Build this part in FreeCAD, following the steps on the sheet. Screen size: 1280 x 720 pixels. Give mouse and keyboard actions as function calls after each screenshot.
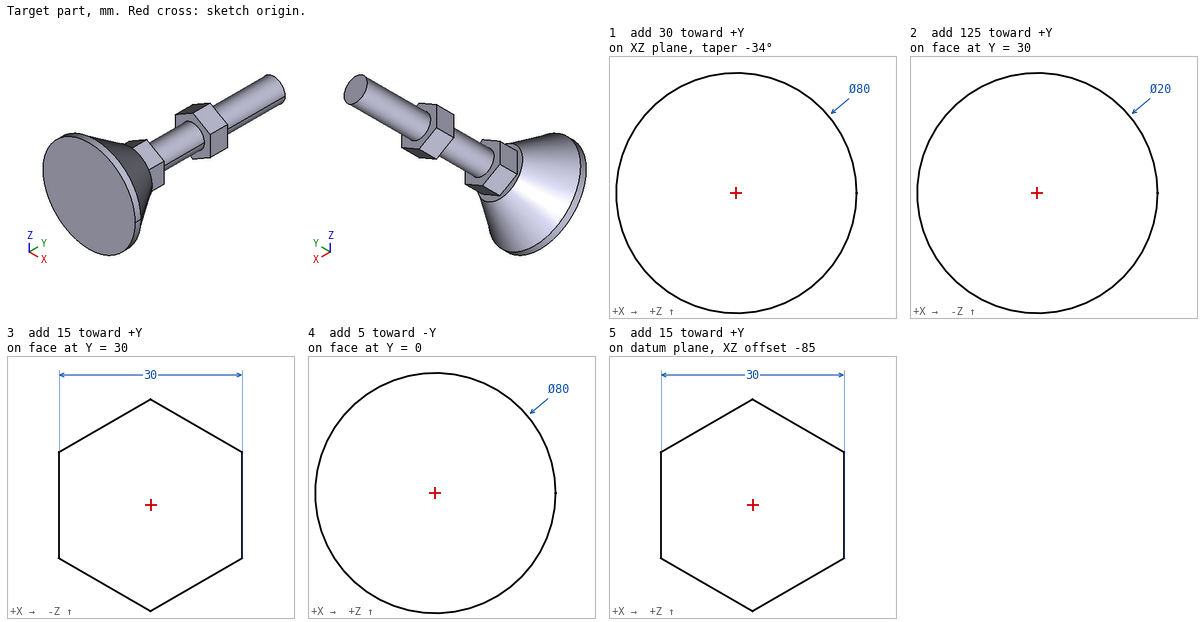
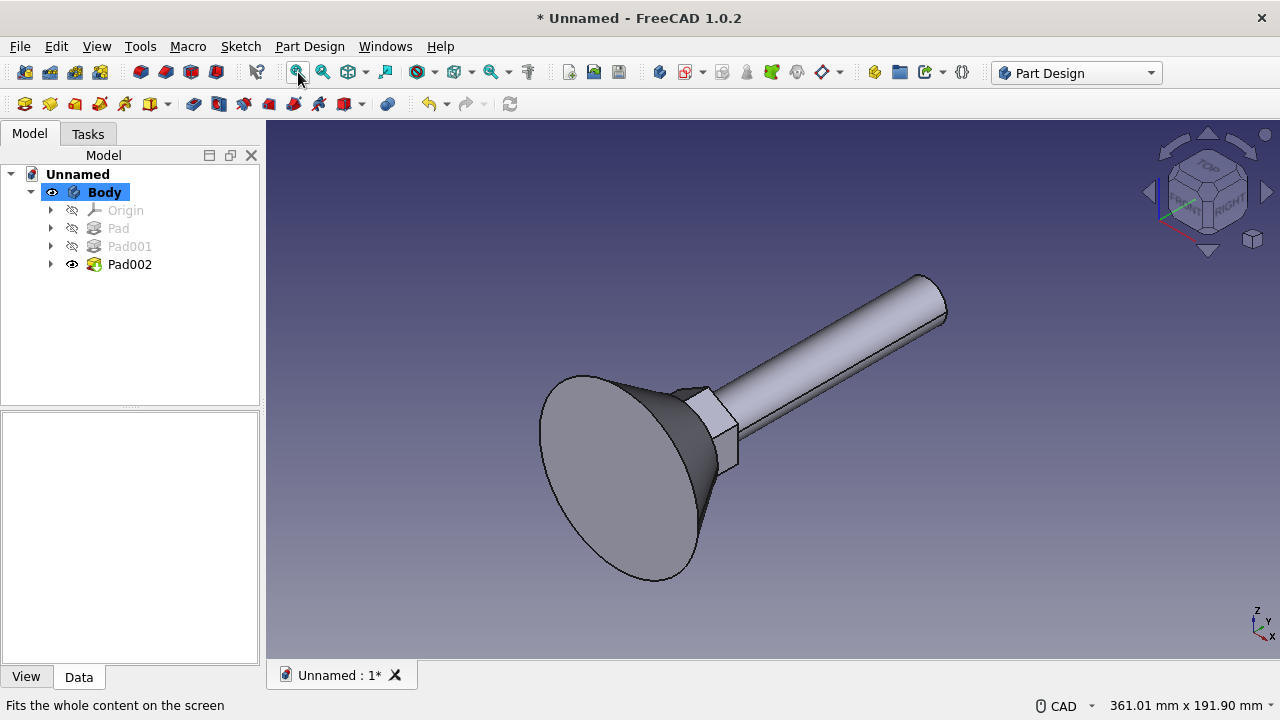
click(619, 477)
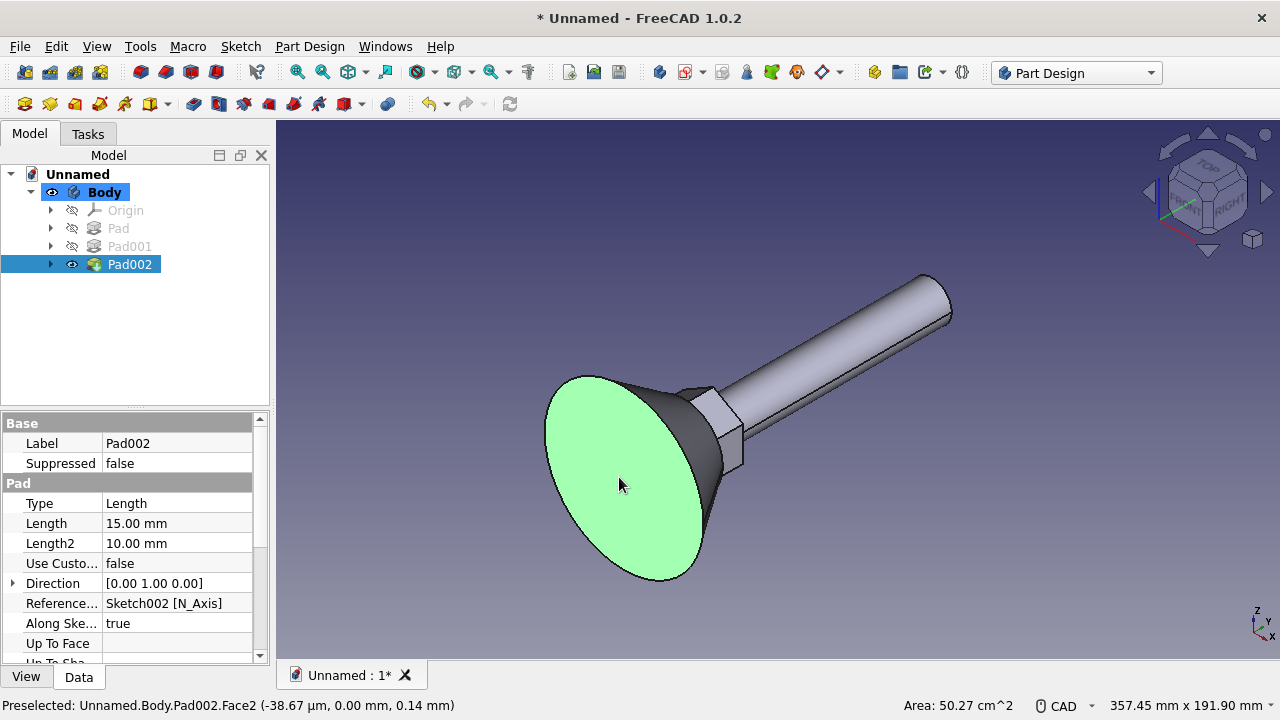
click(684, 72)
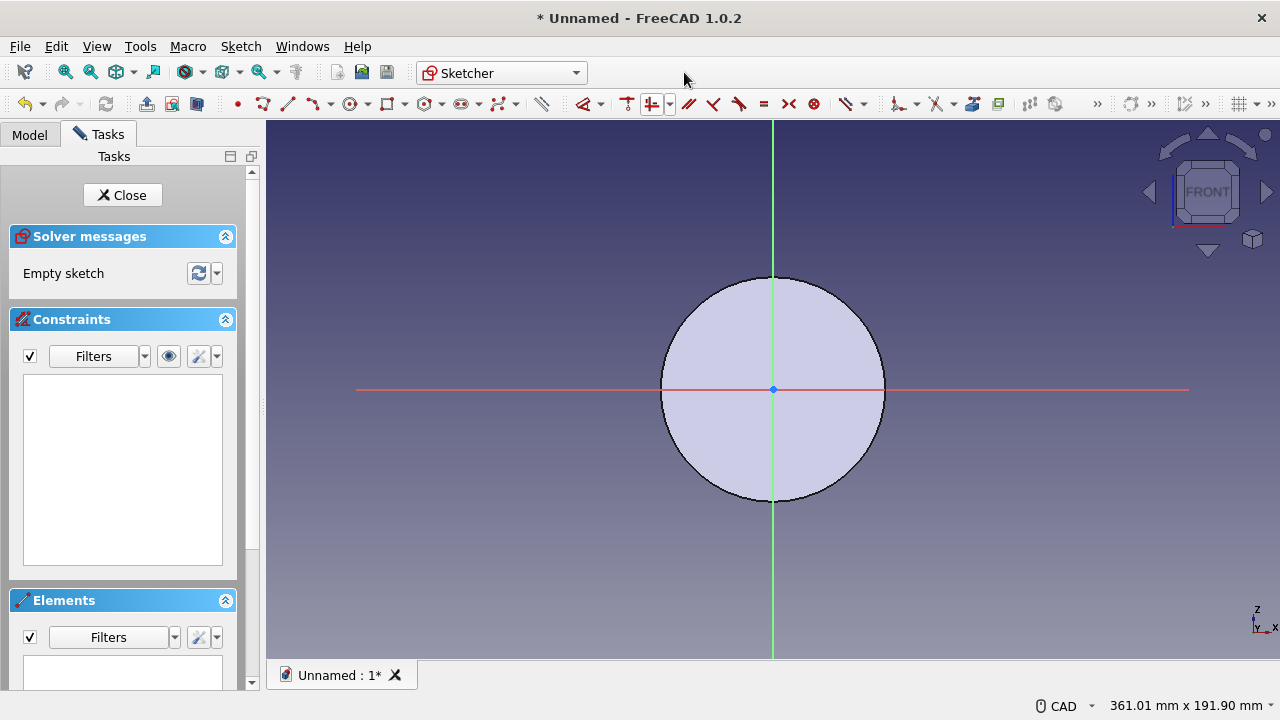
scroll(912, 390, up, 2)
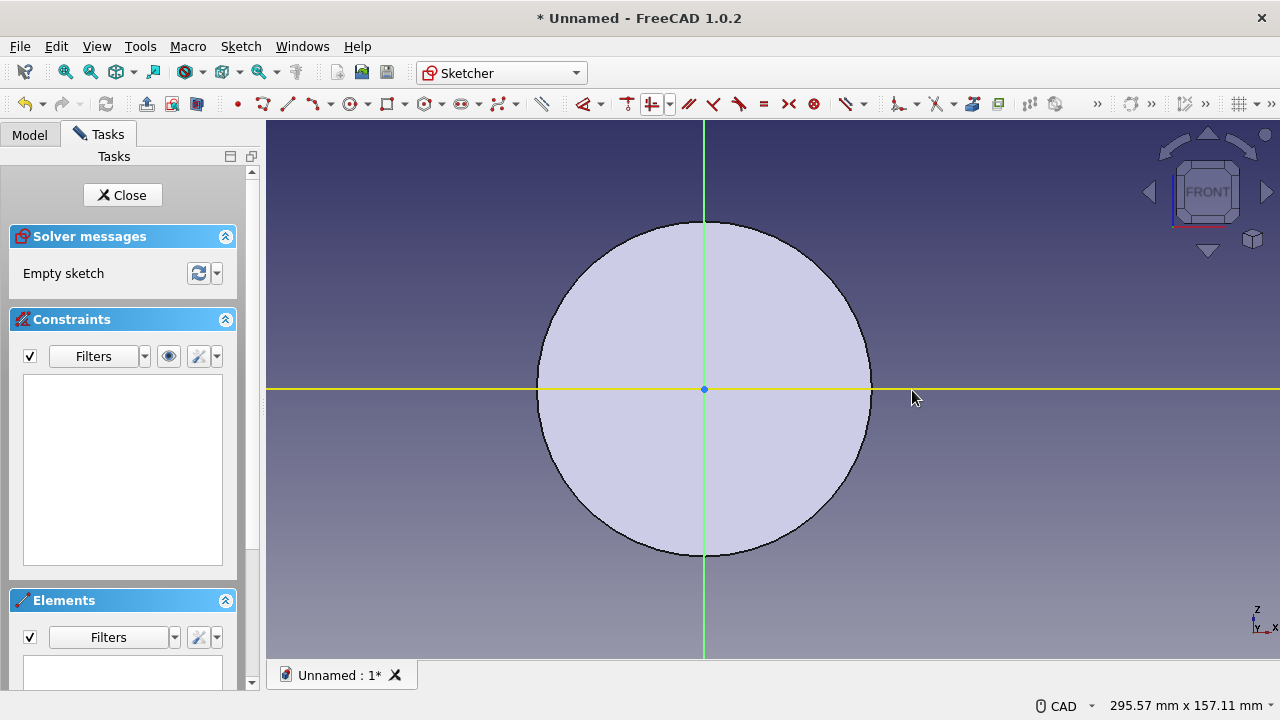
click(350, 104)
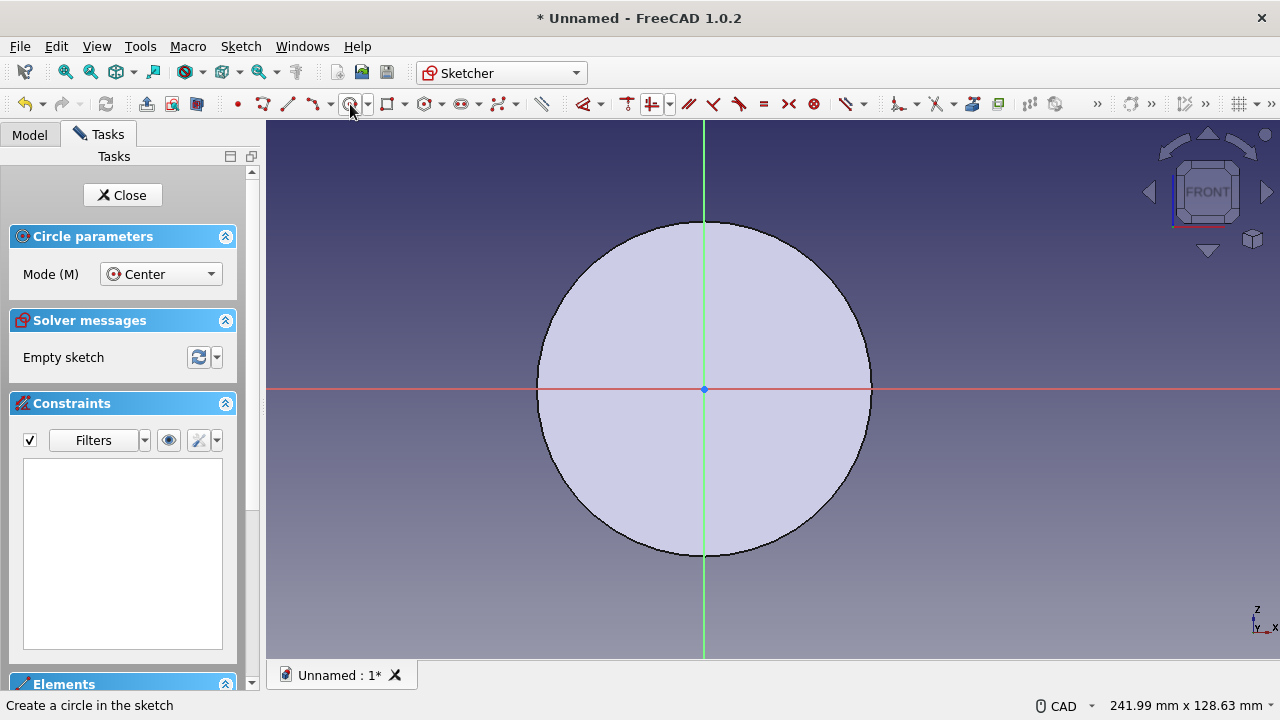
click(704, 389)
move(823, 270)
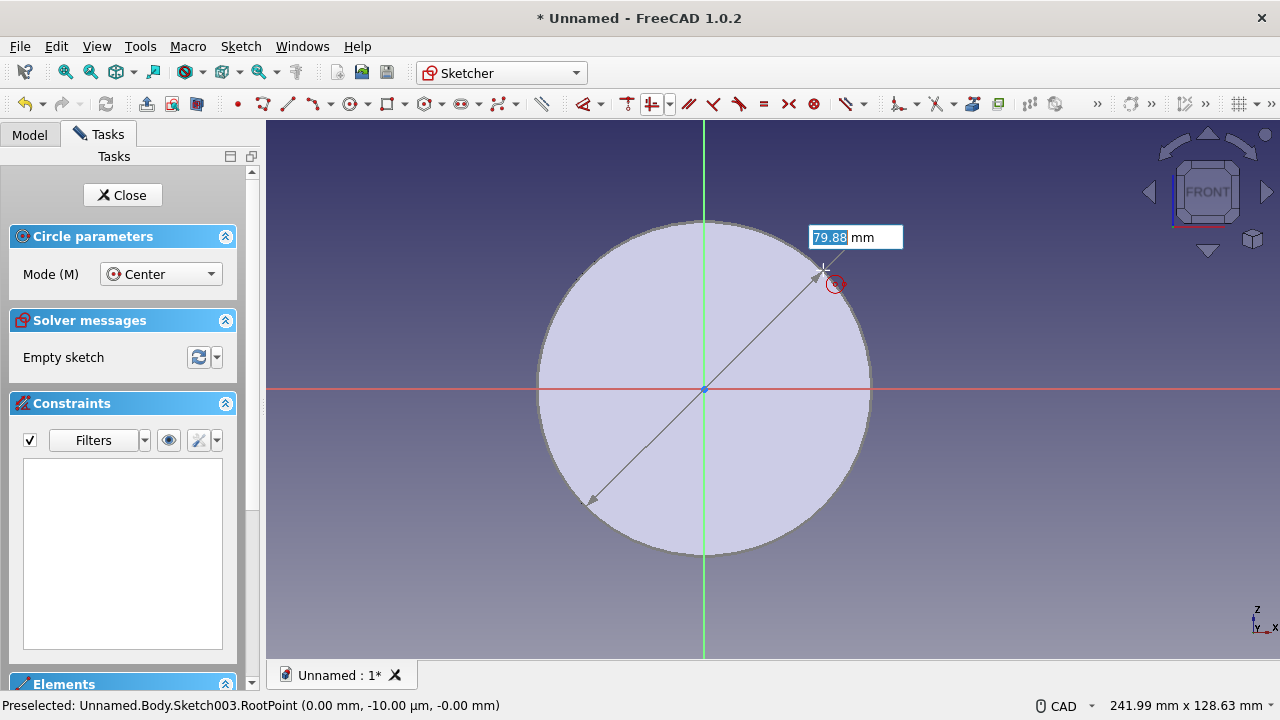
text(80)
key(Return)
key(Escape)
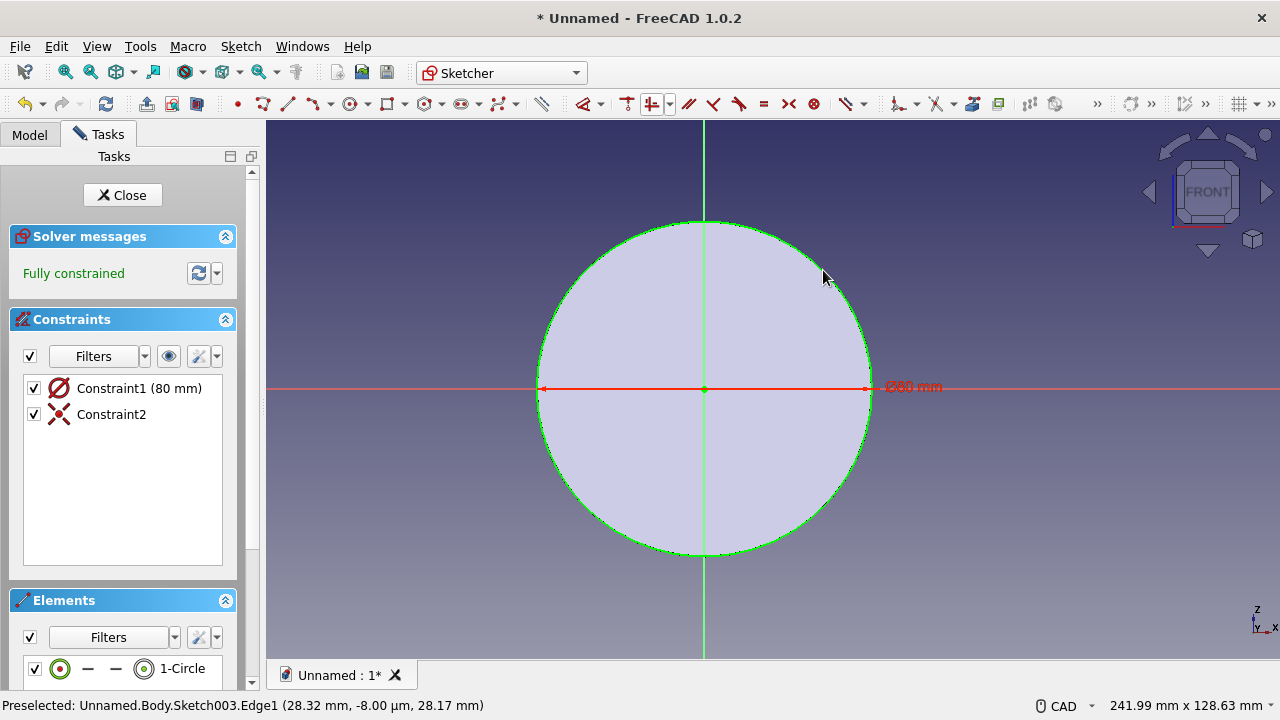
click(123, 195)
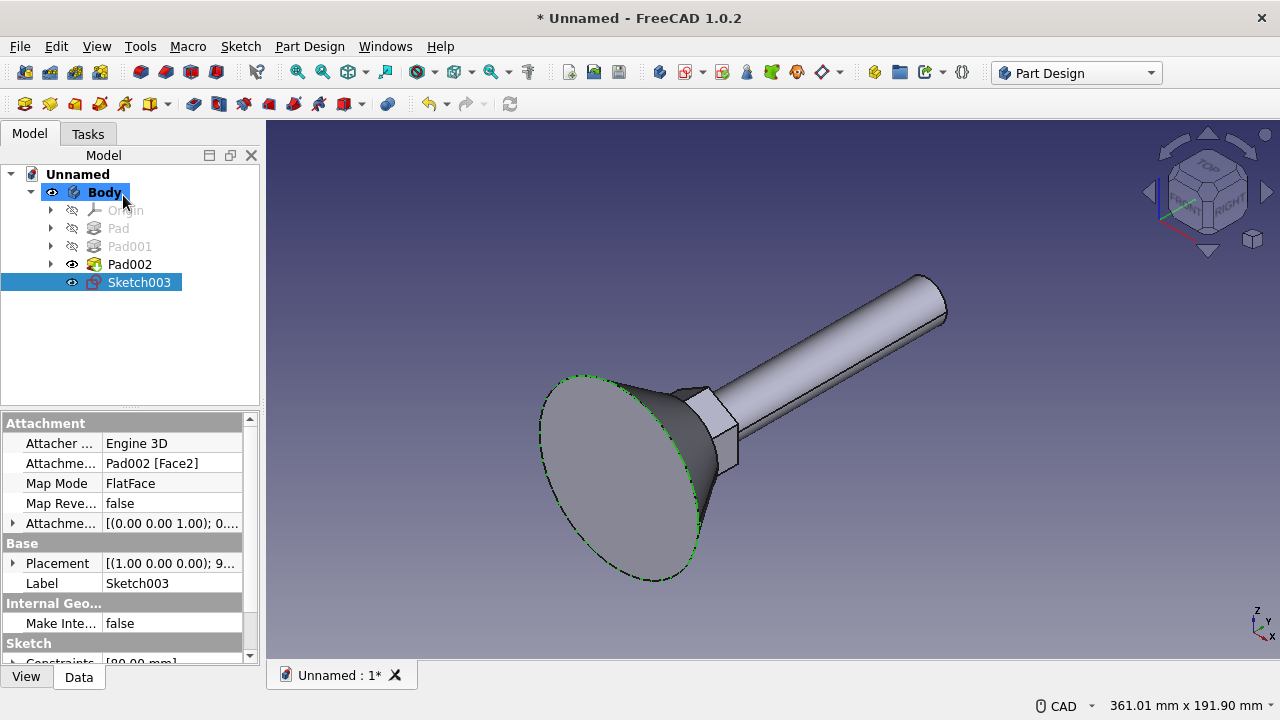
click(25, 104)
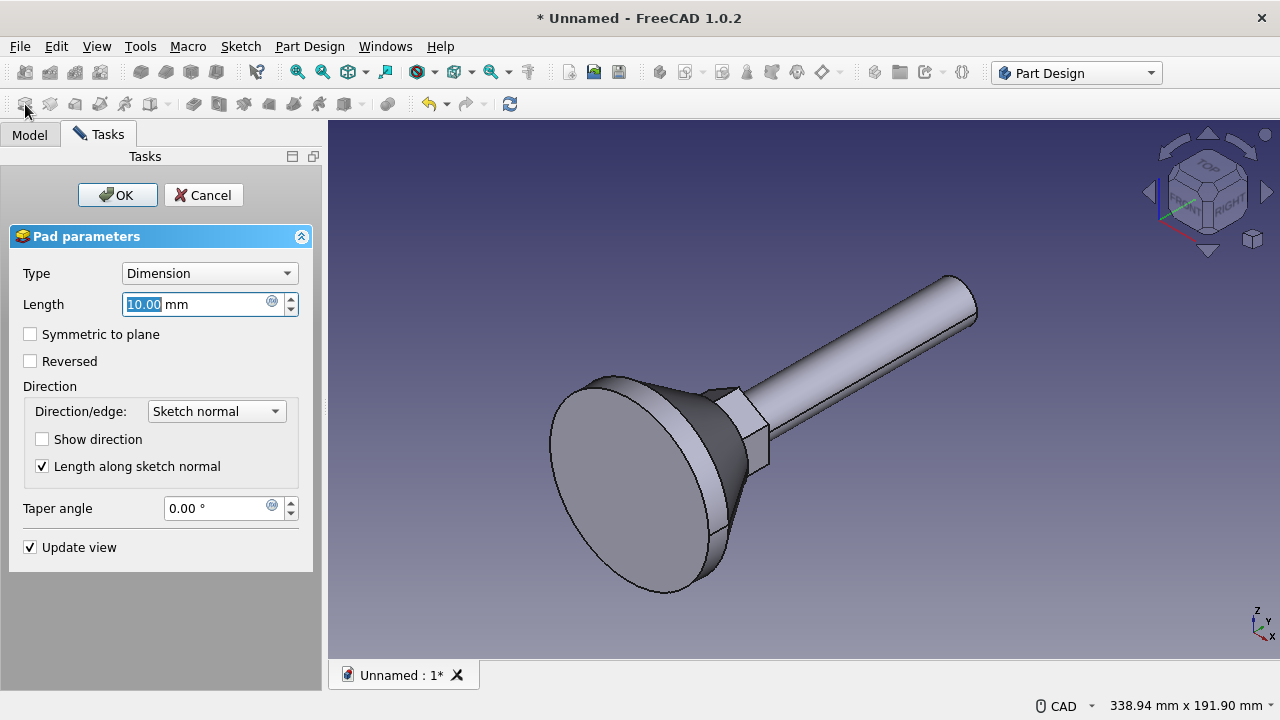
text(5)
key(Tab)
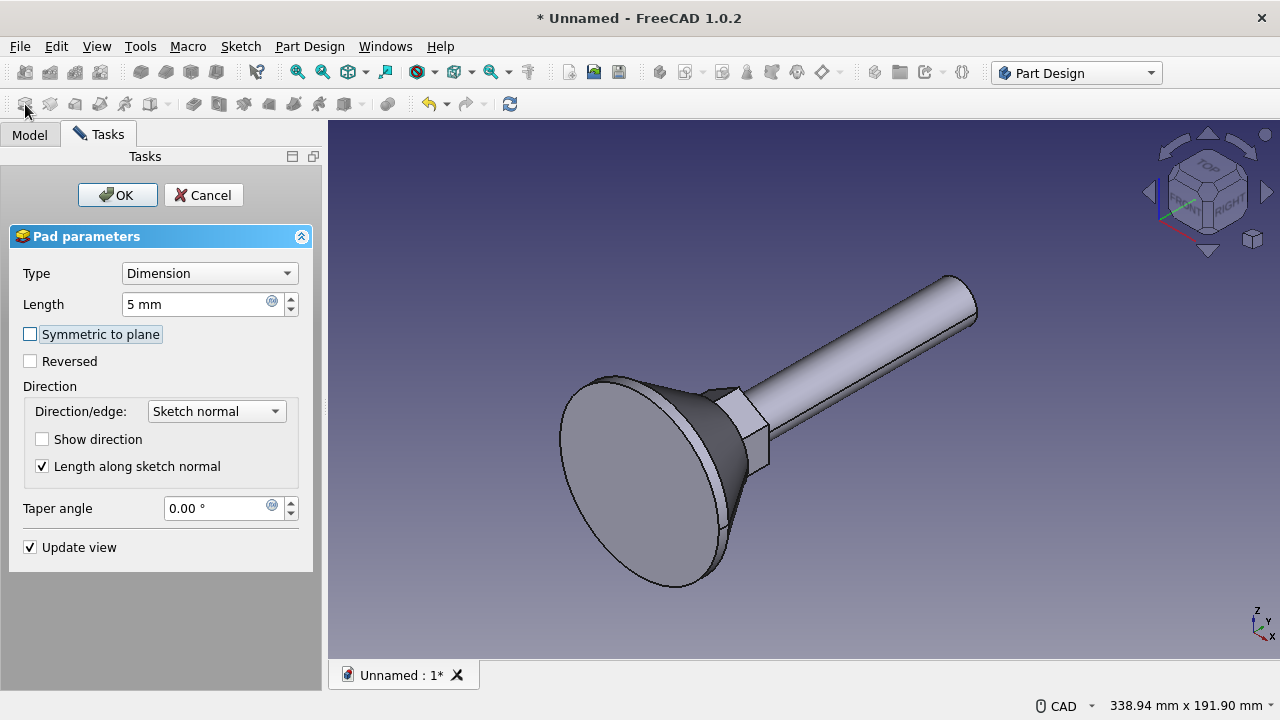
click(118, 195)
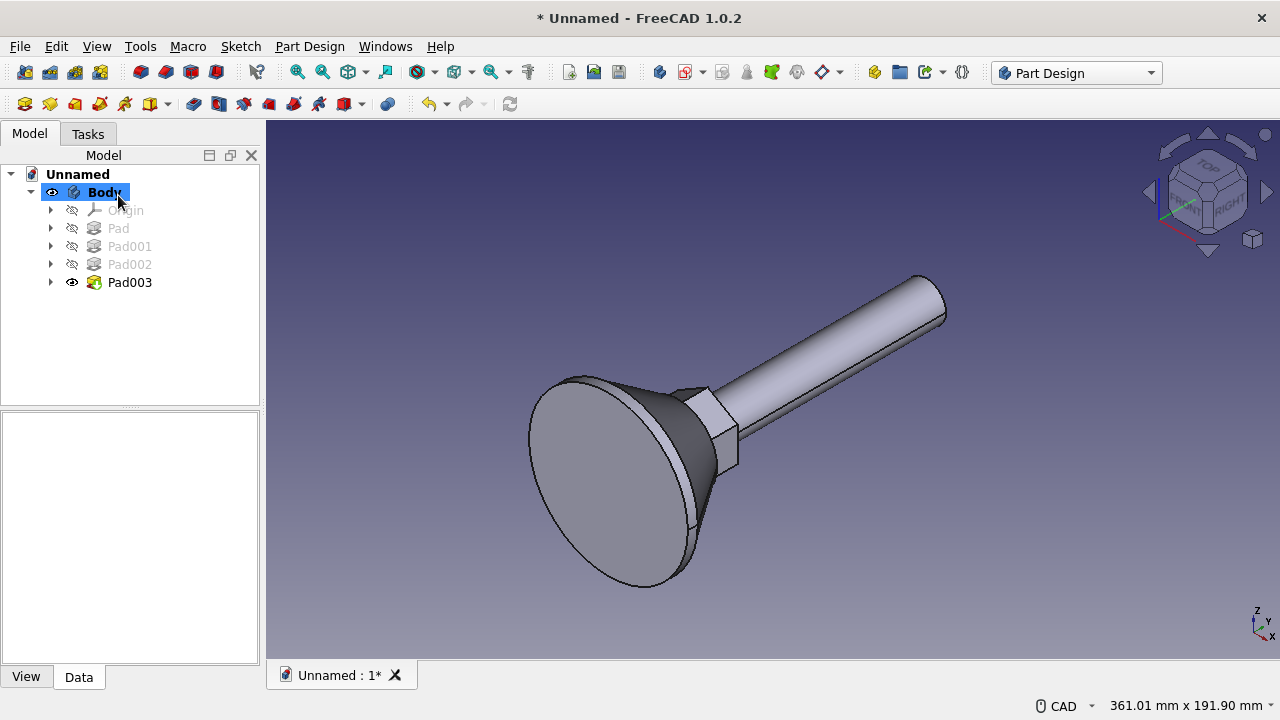
click(51, 210)